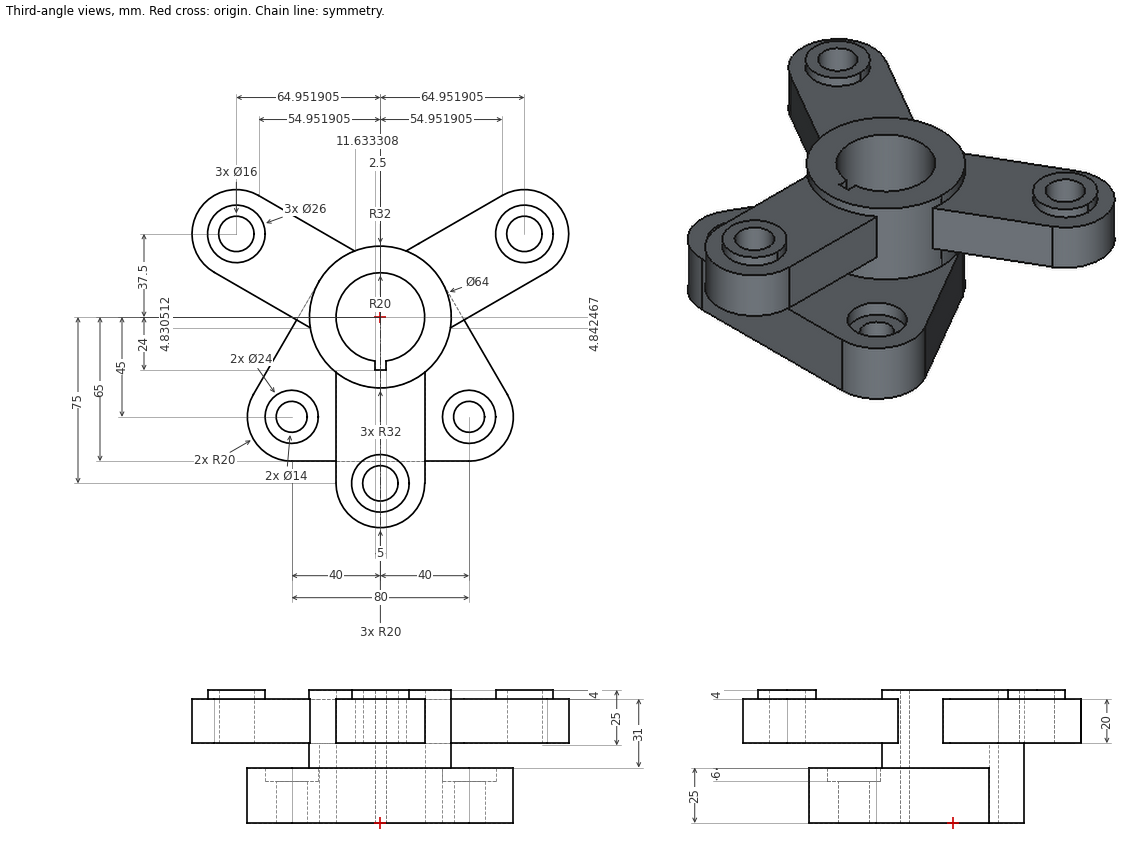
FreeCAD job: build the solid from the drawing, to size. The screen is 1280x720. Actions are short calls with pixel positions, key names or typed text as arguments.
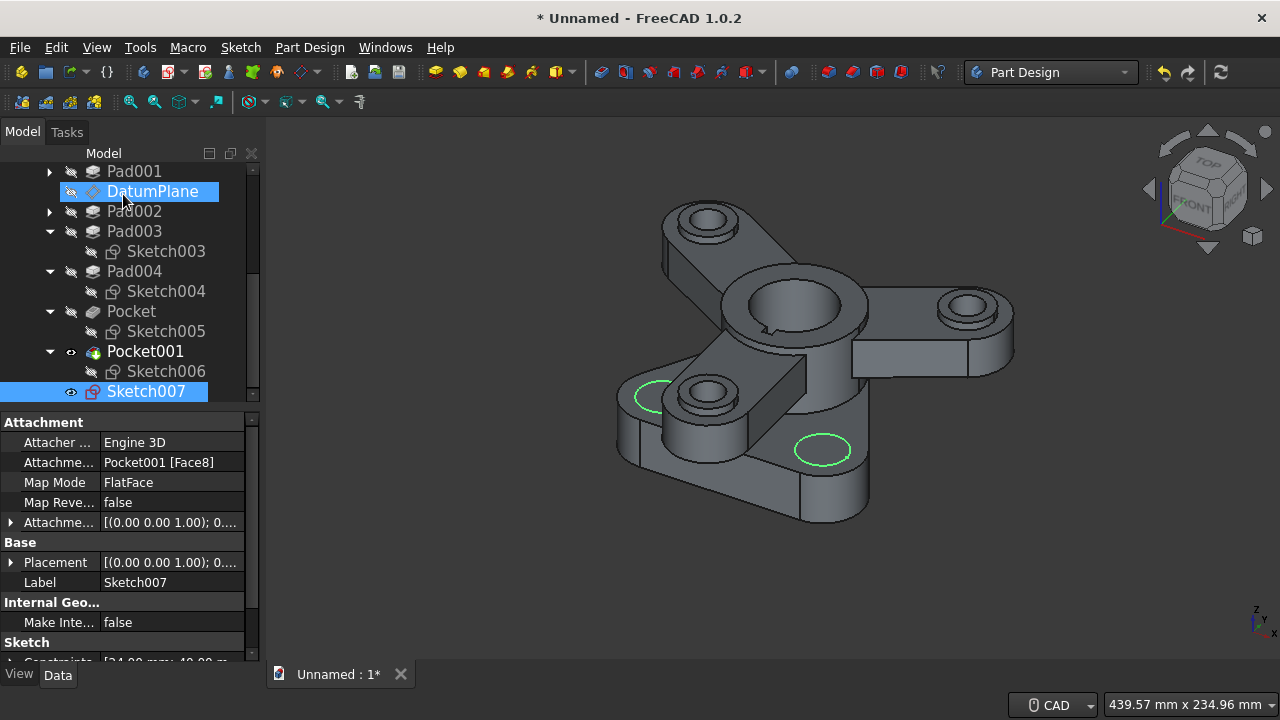
click(602, 72)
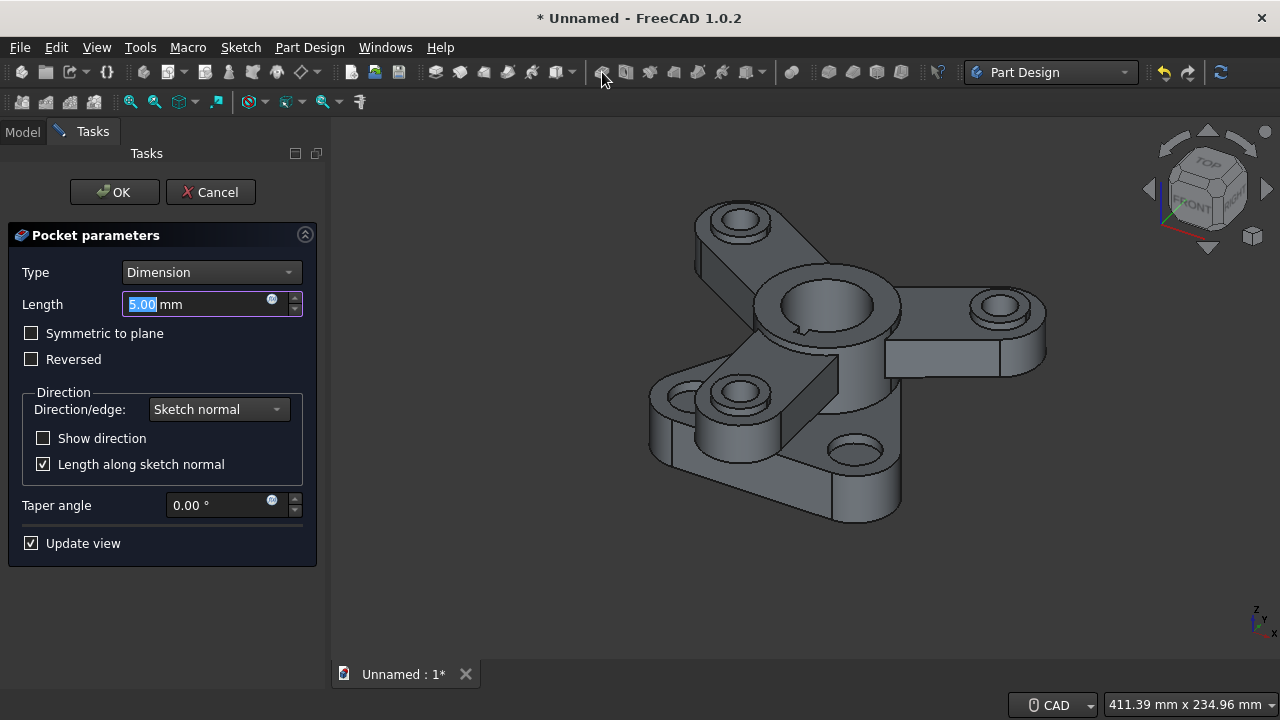
text(6)
key(Tab)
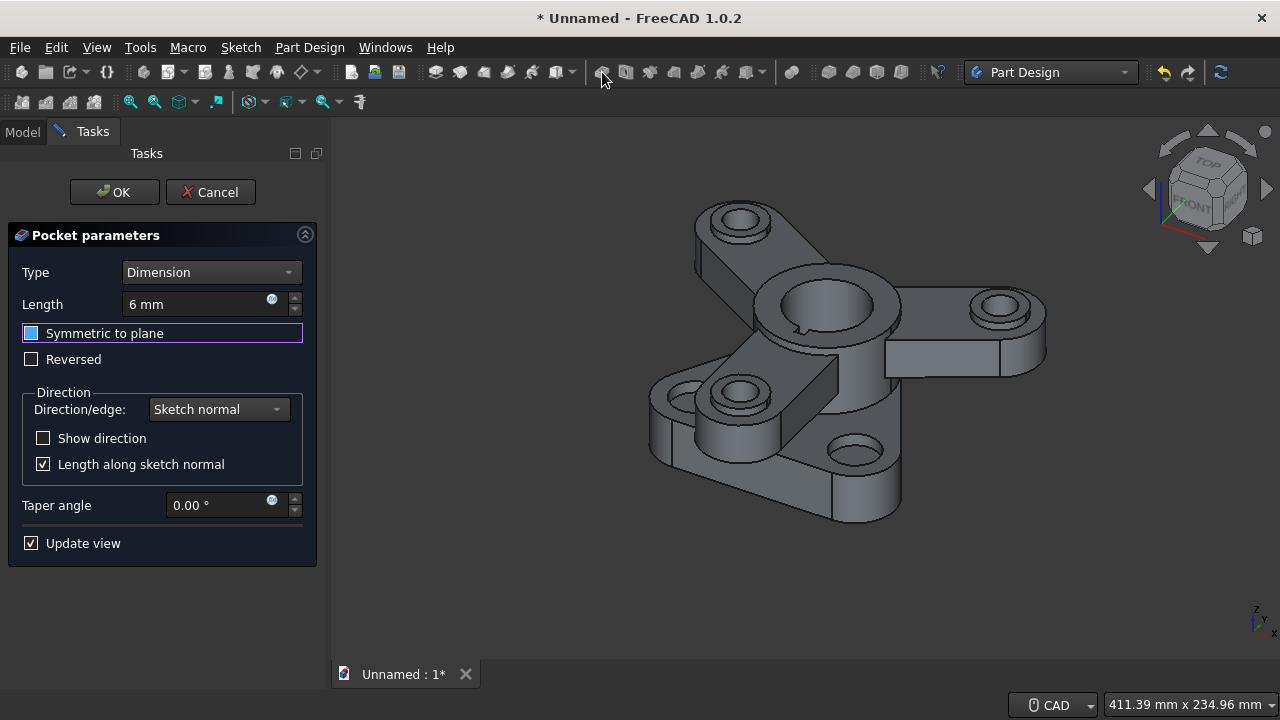
click(115, 192)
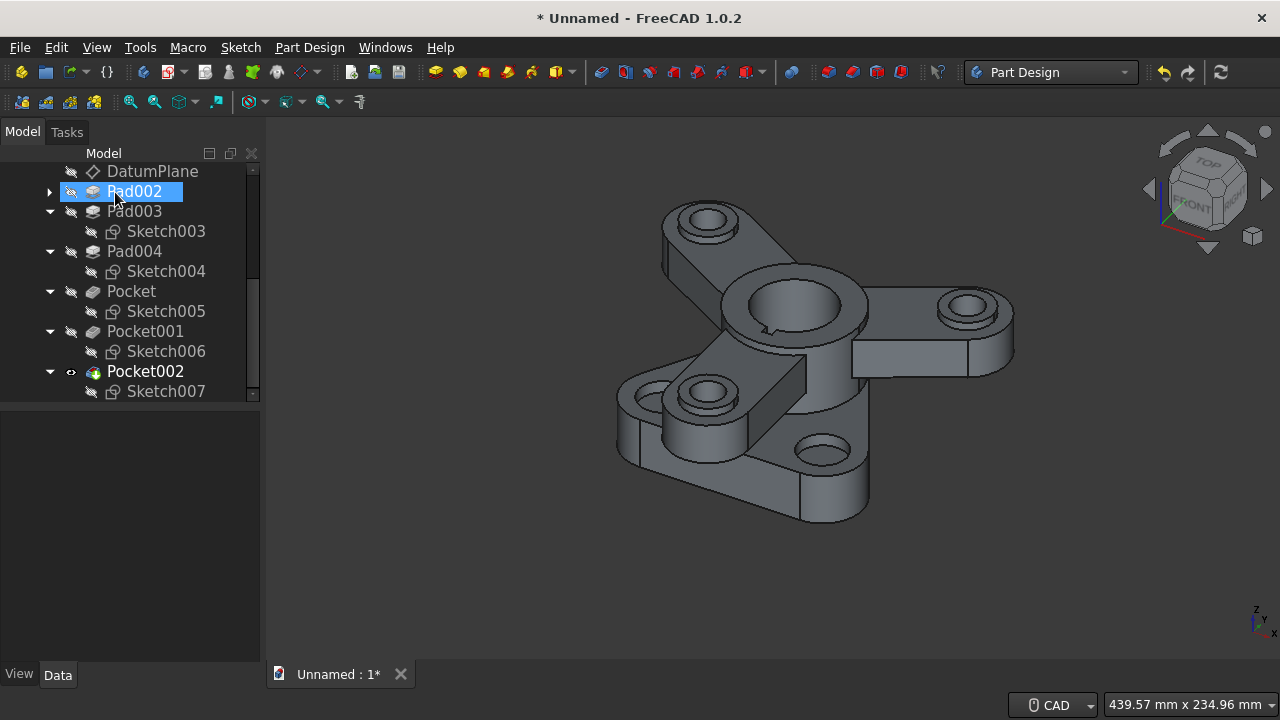
click(827, 456)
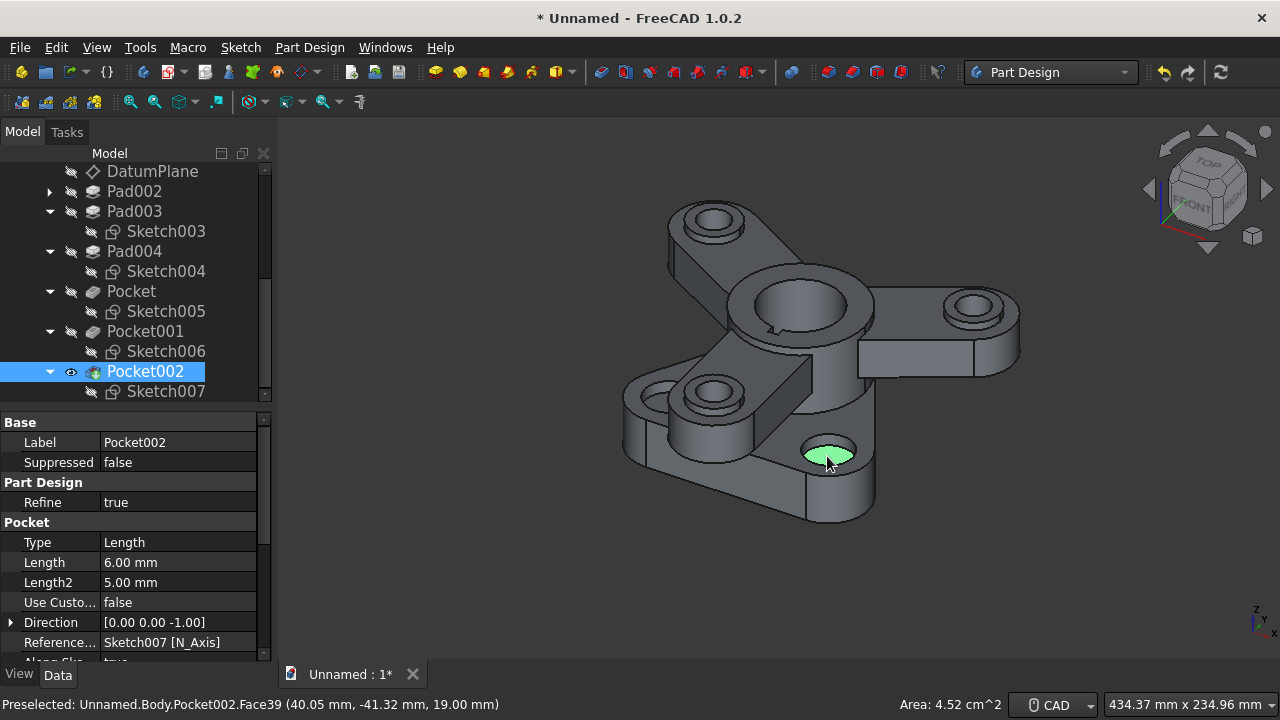
click(168, 72)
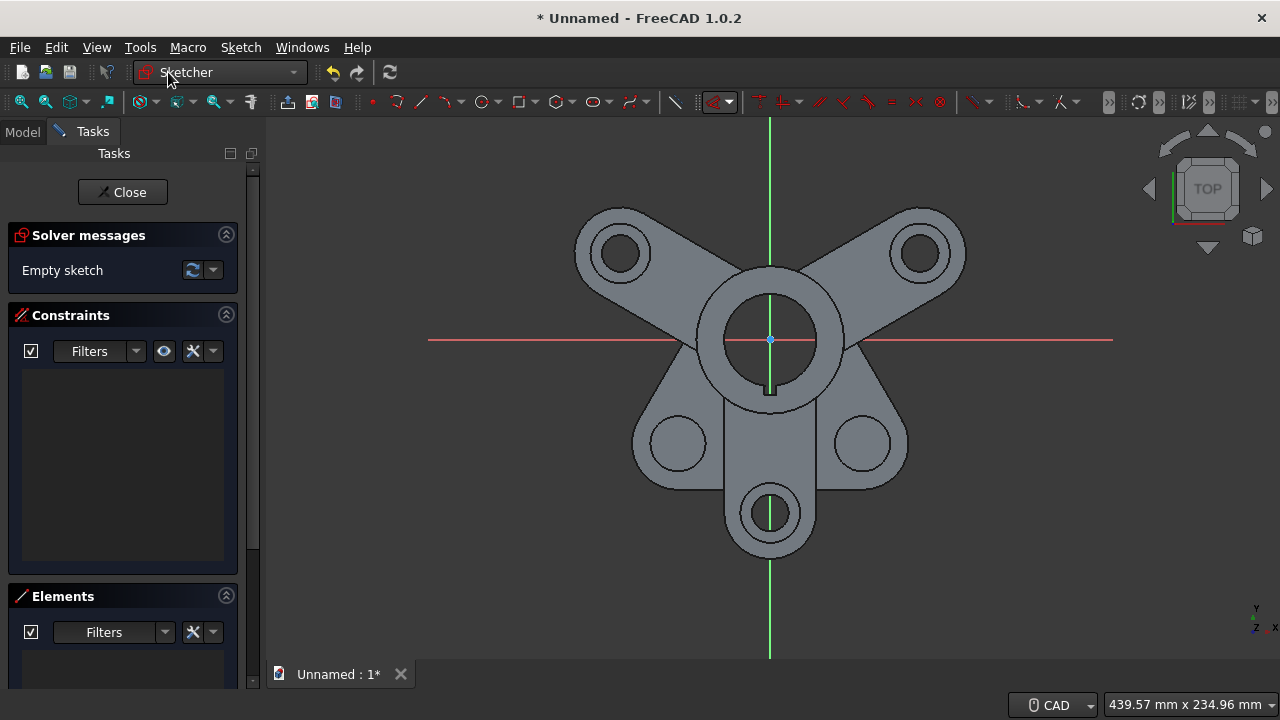
key(q)
key(s)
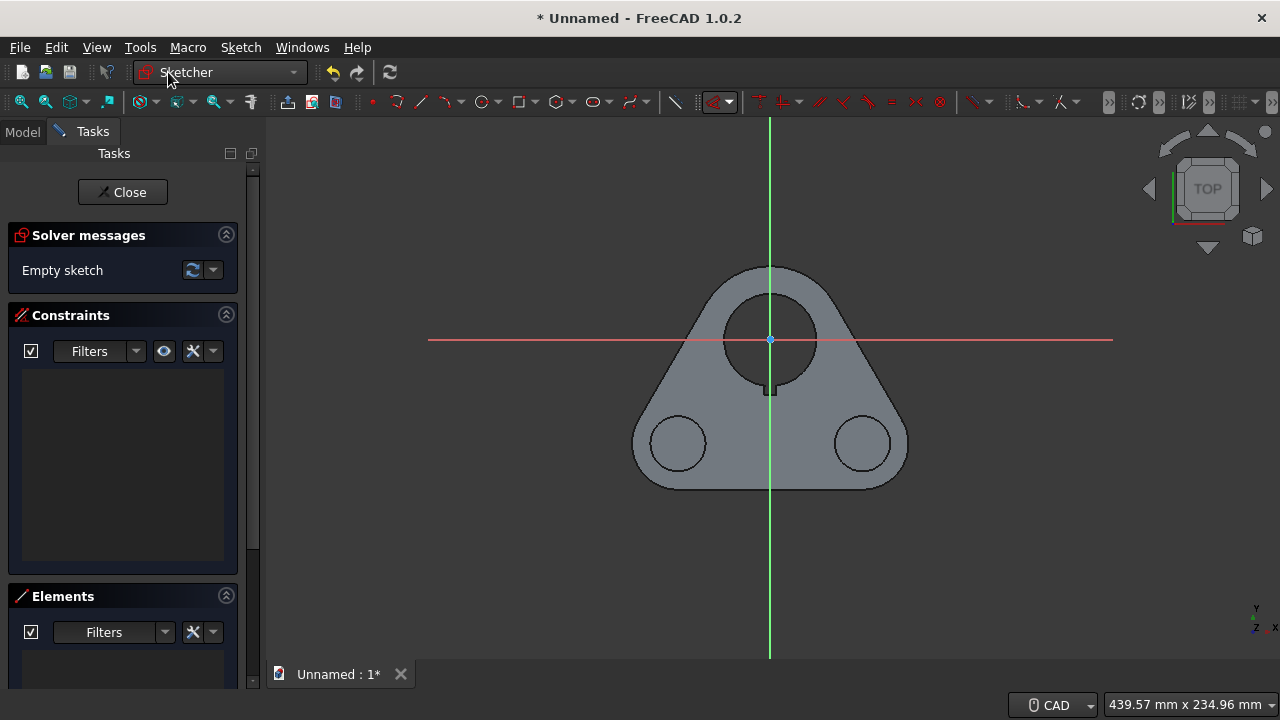
scroll(809, 407, up, 5)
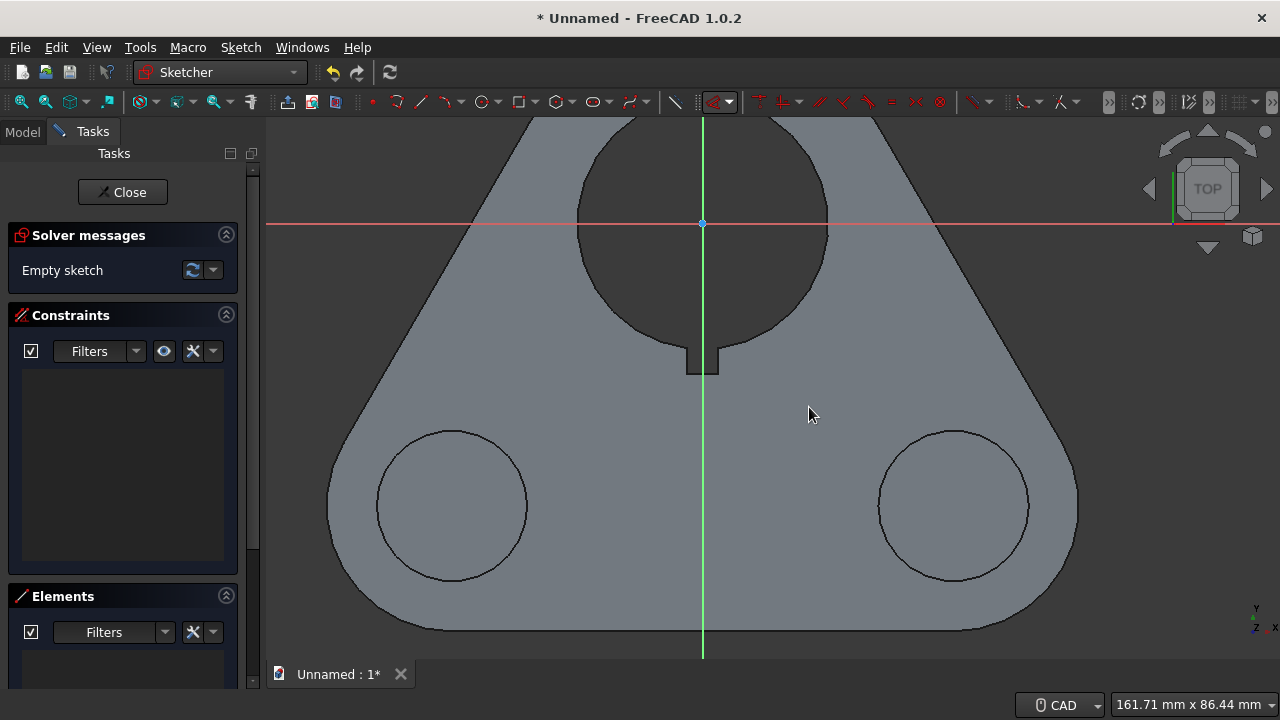
click(482, 102)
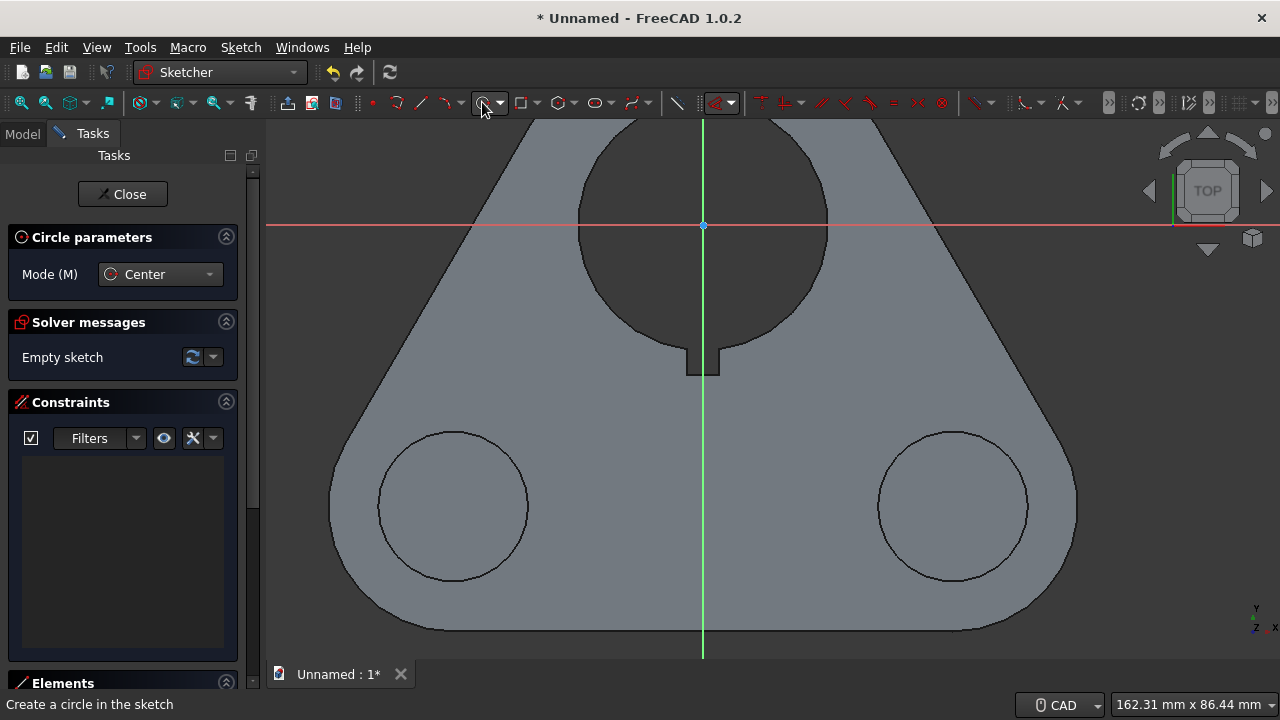
click(453, 507)
click(484, 476)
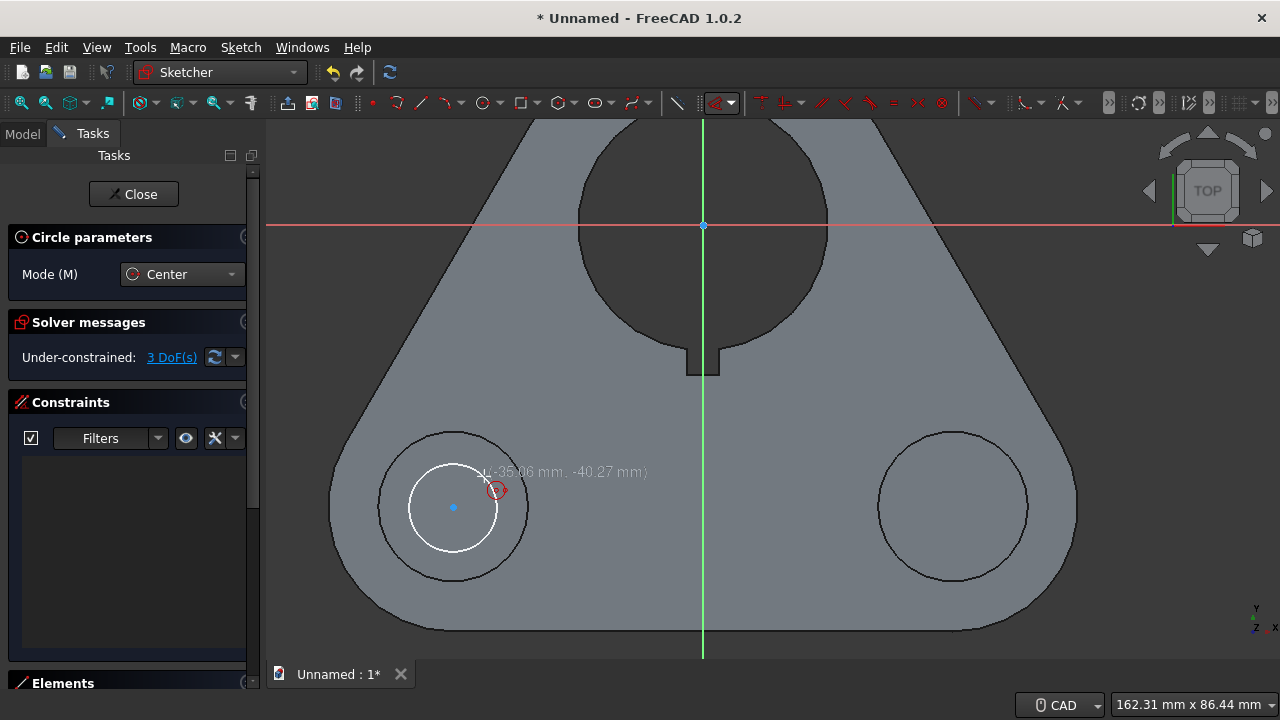
click(953, 507)
click(984, 476)
key(Escape)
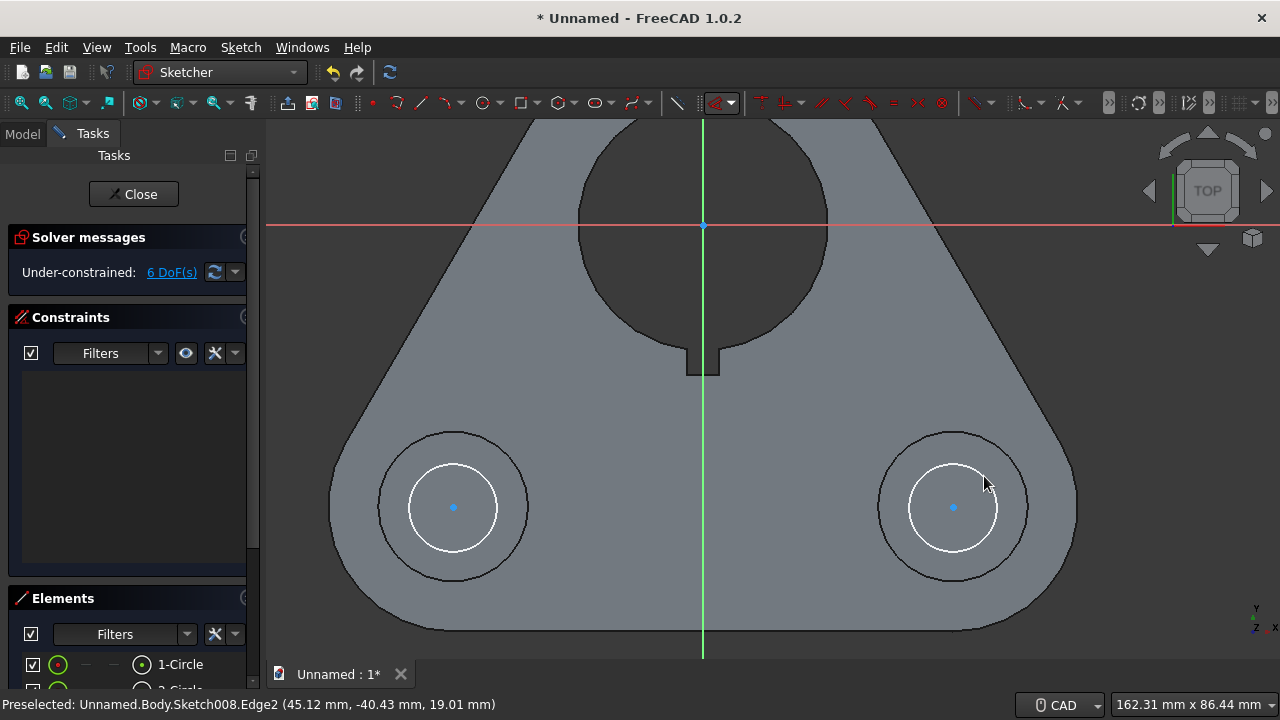
click(484, 477)